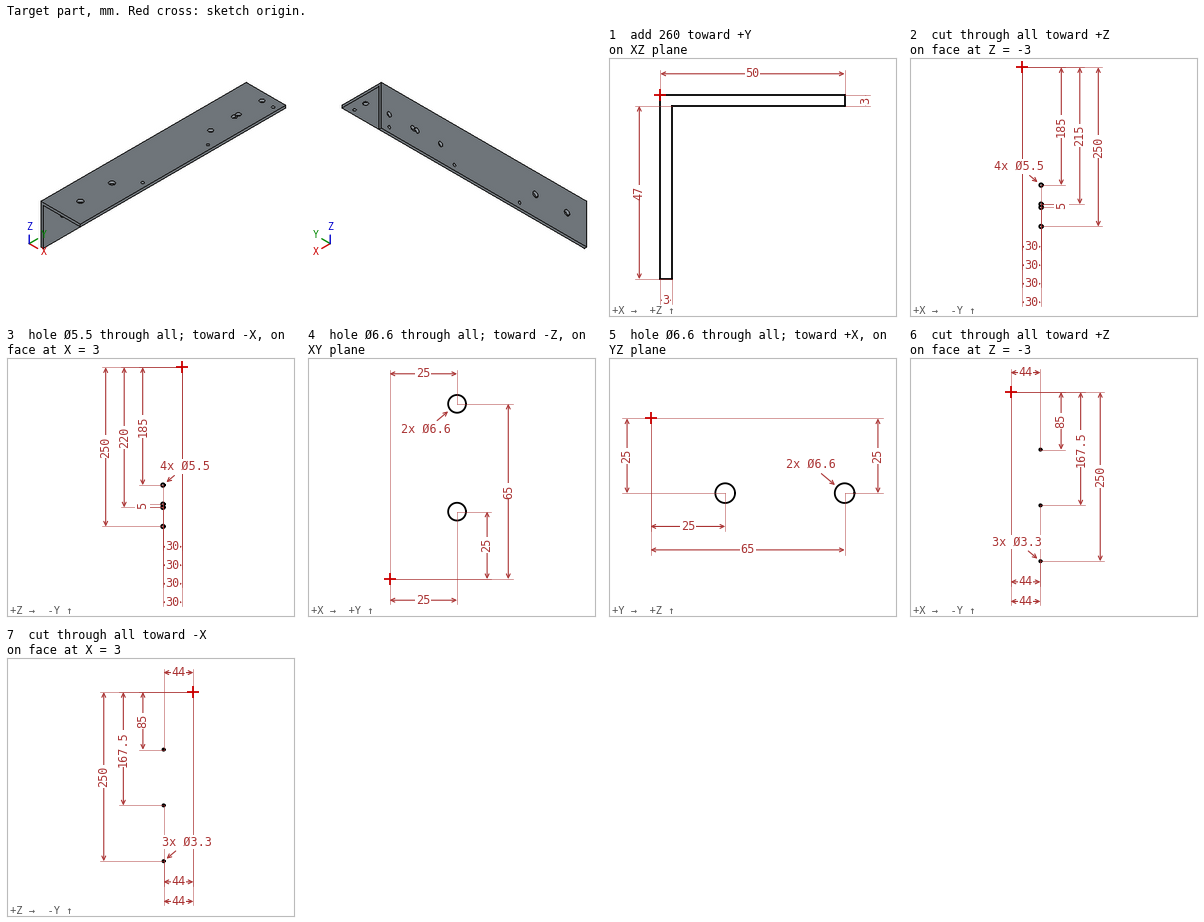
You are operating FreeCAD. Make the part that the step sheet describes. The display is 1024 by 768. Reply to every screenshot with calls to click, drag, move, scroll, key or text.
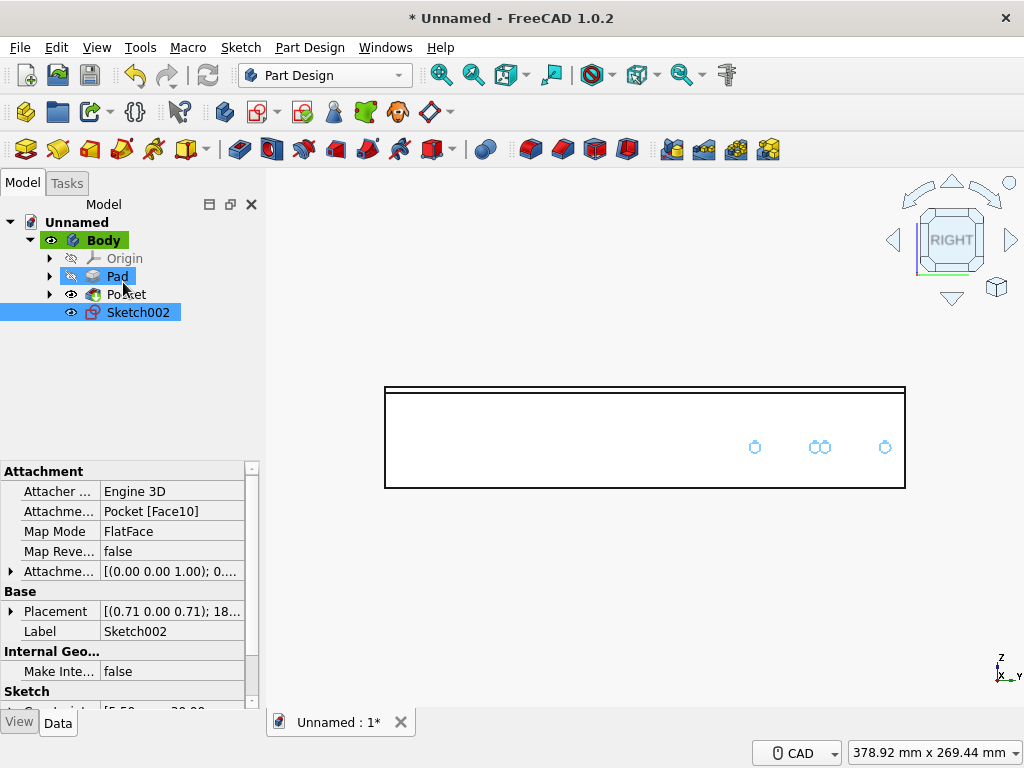
click(272, 150)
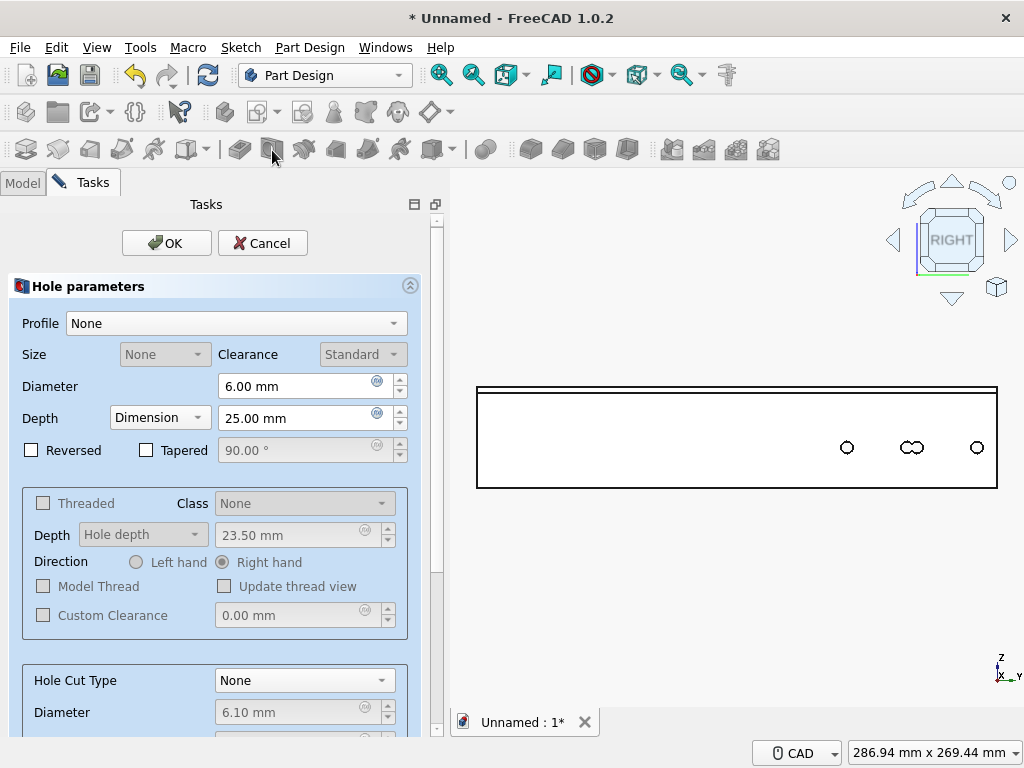
triple_click(305, 386)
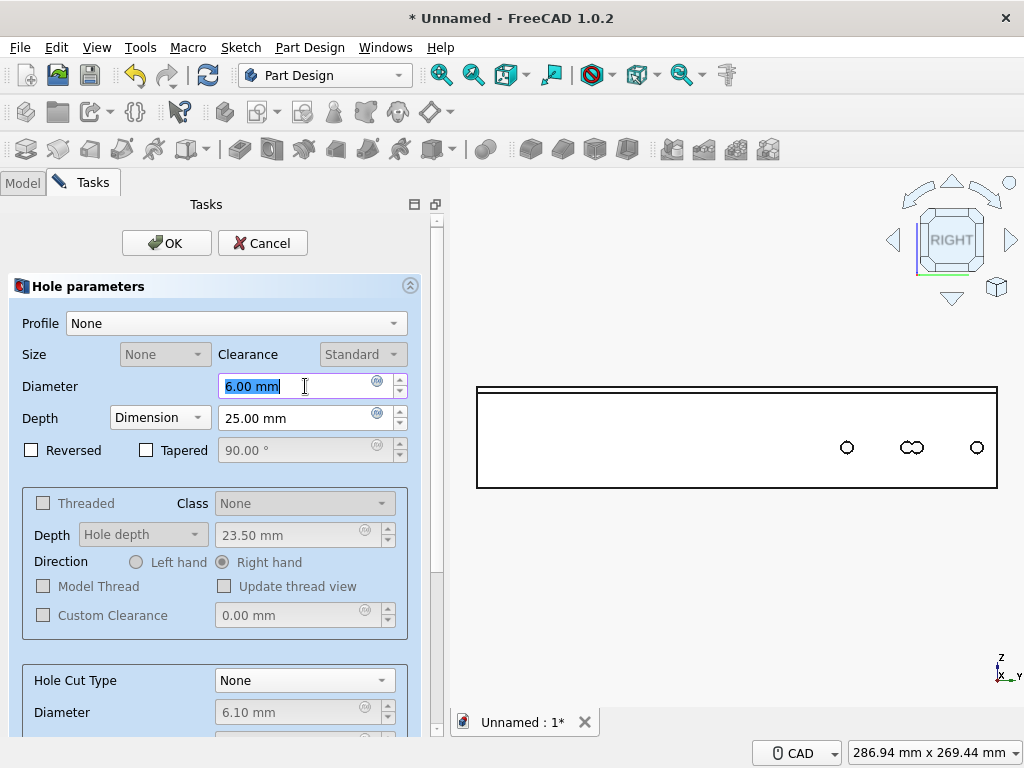
text(5.5)
key(Tab)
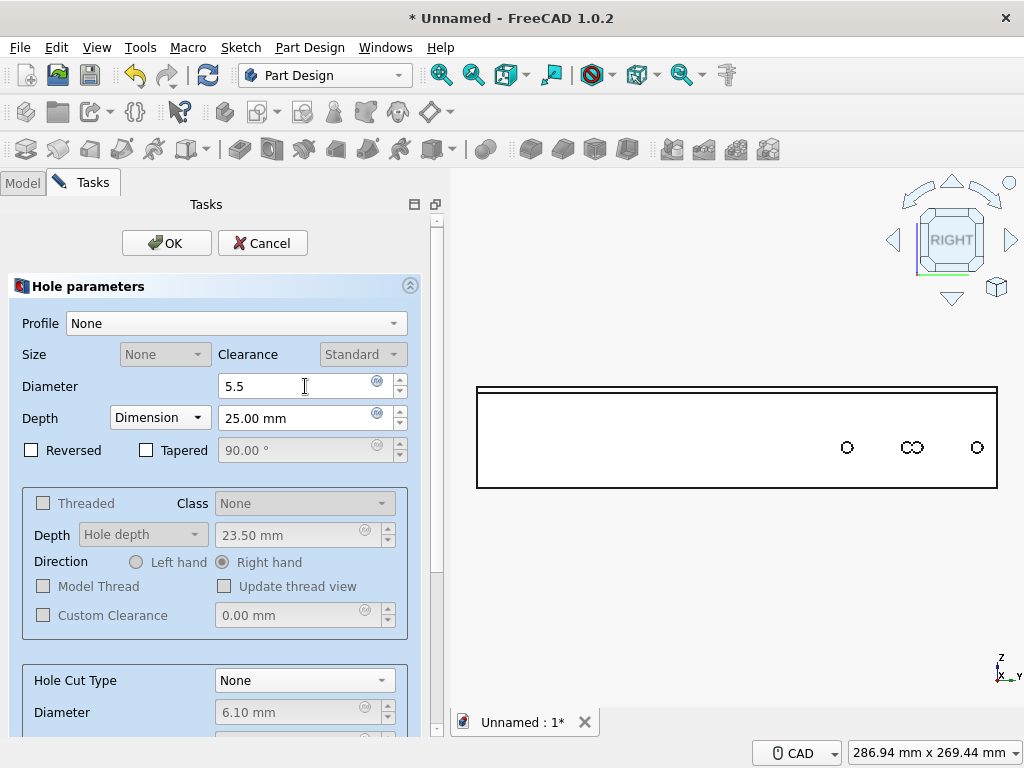
click(161, 418)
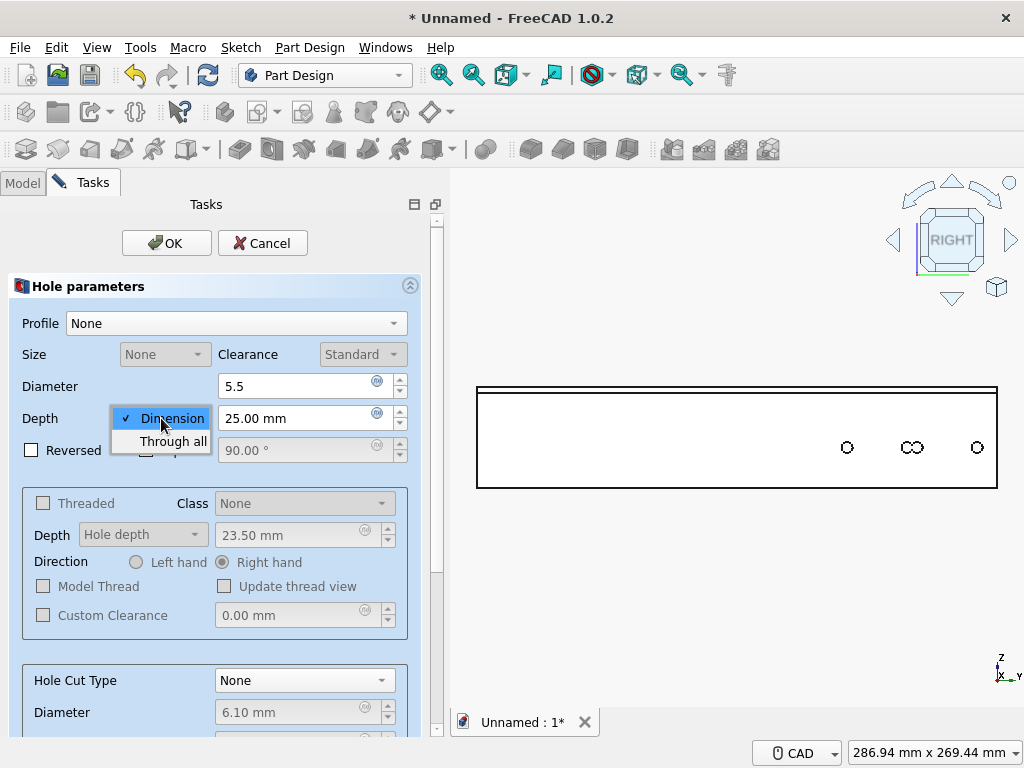
click(160, 442)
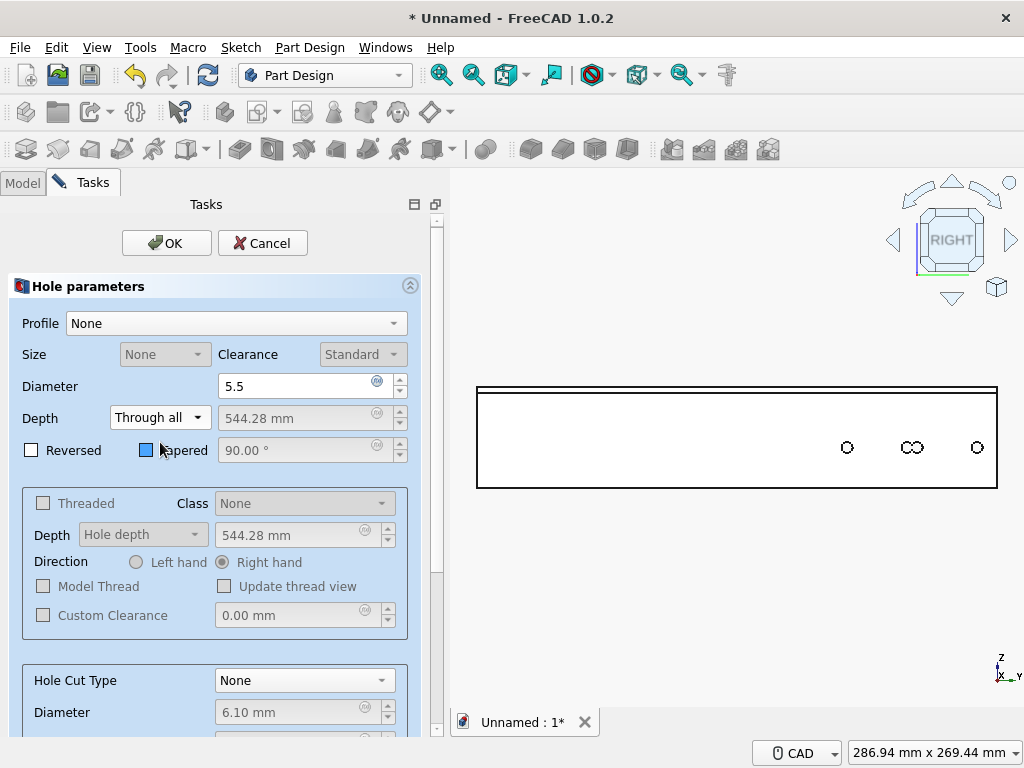
click(167, 243)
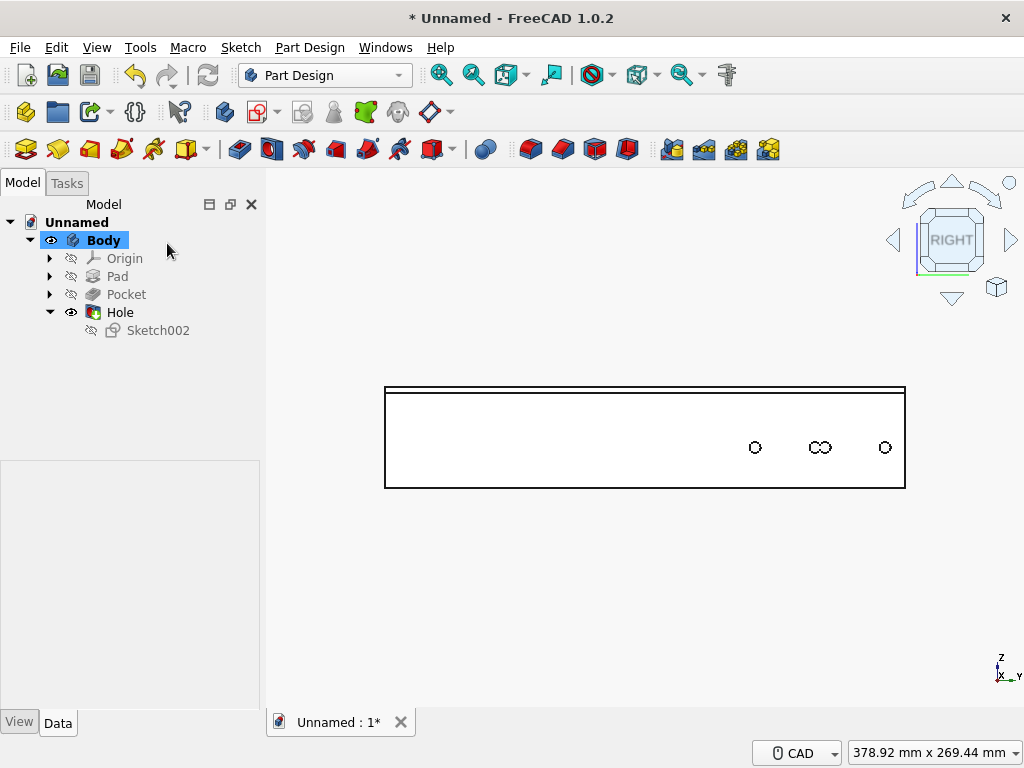
click(258, 112)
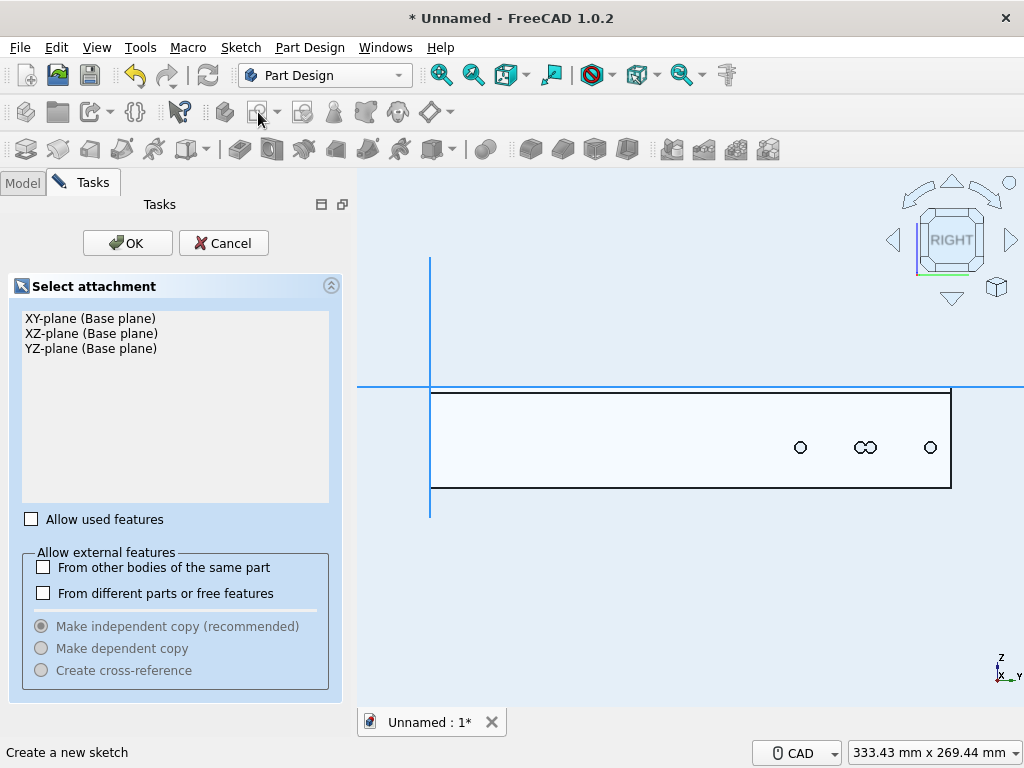
click(82, 318)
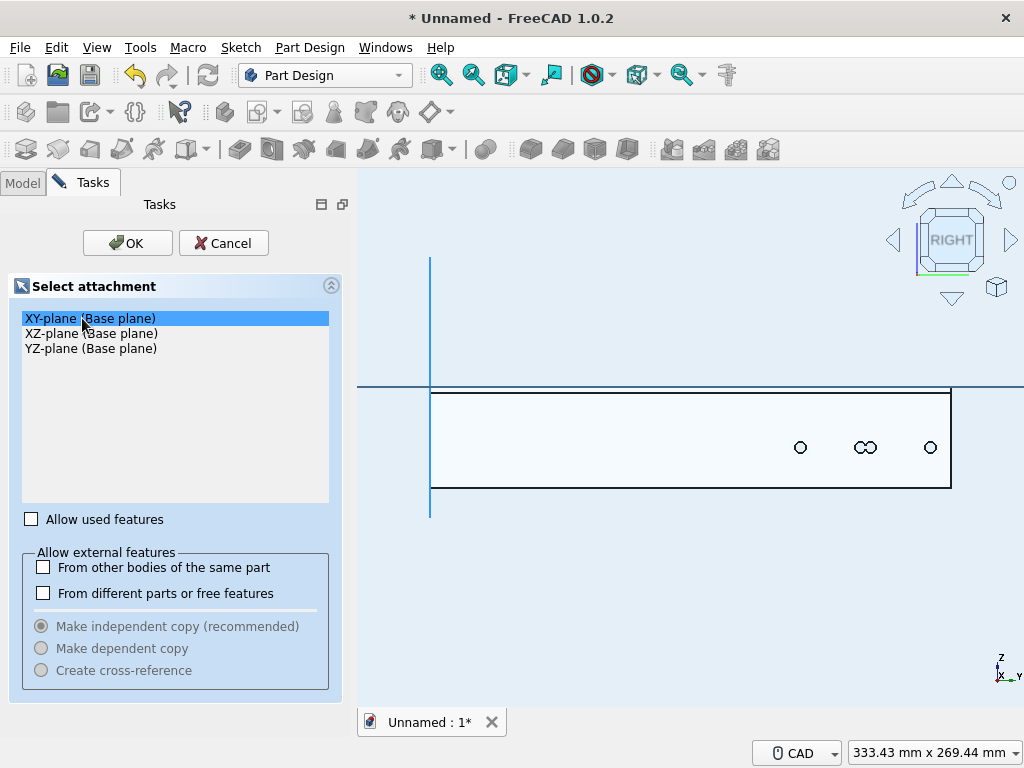
click(128, 243)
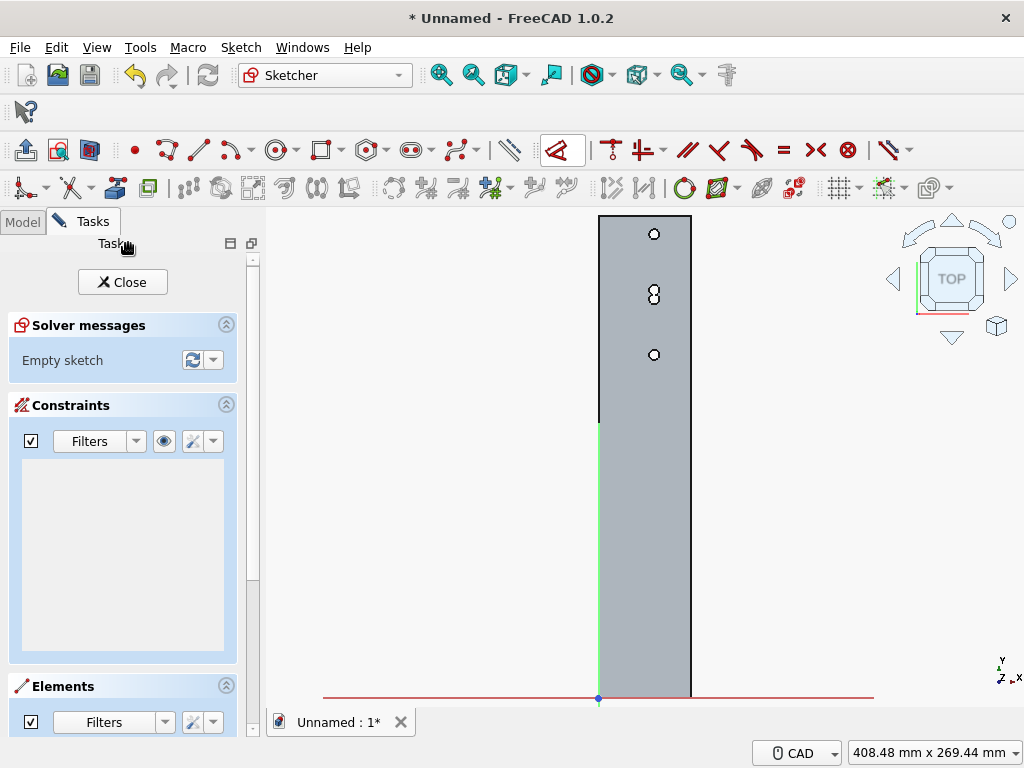
scroll(576, 457, down, 5)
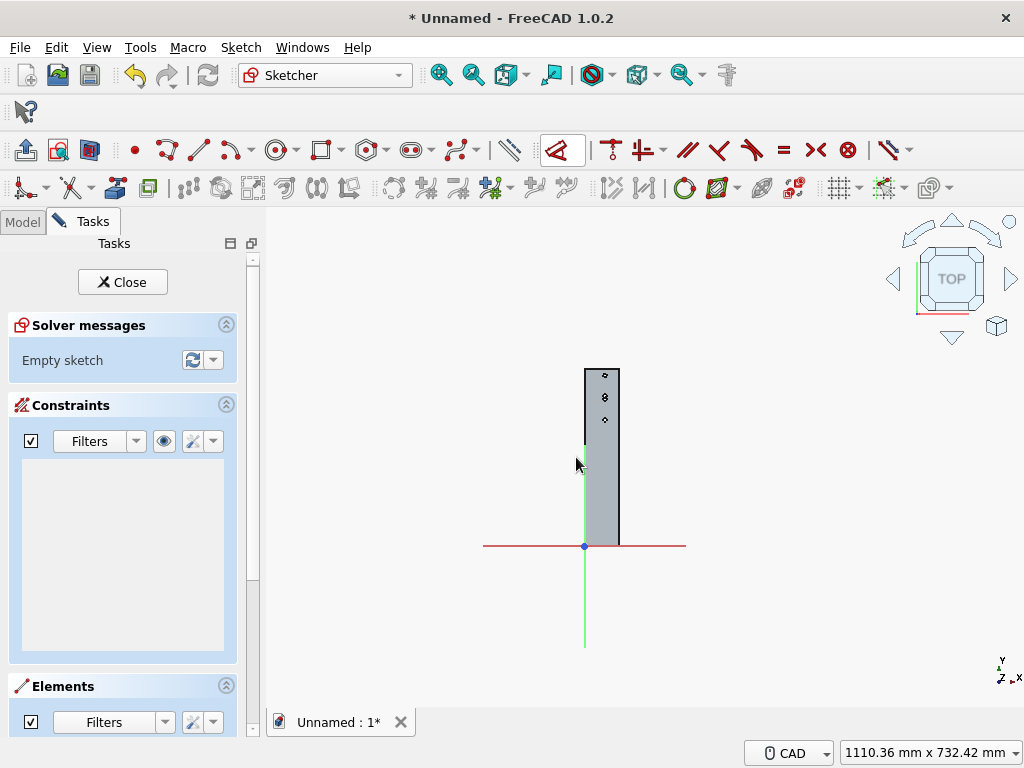
scroll(597, 533, up, 10)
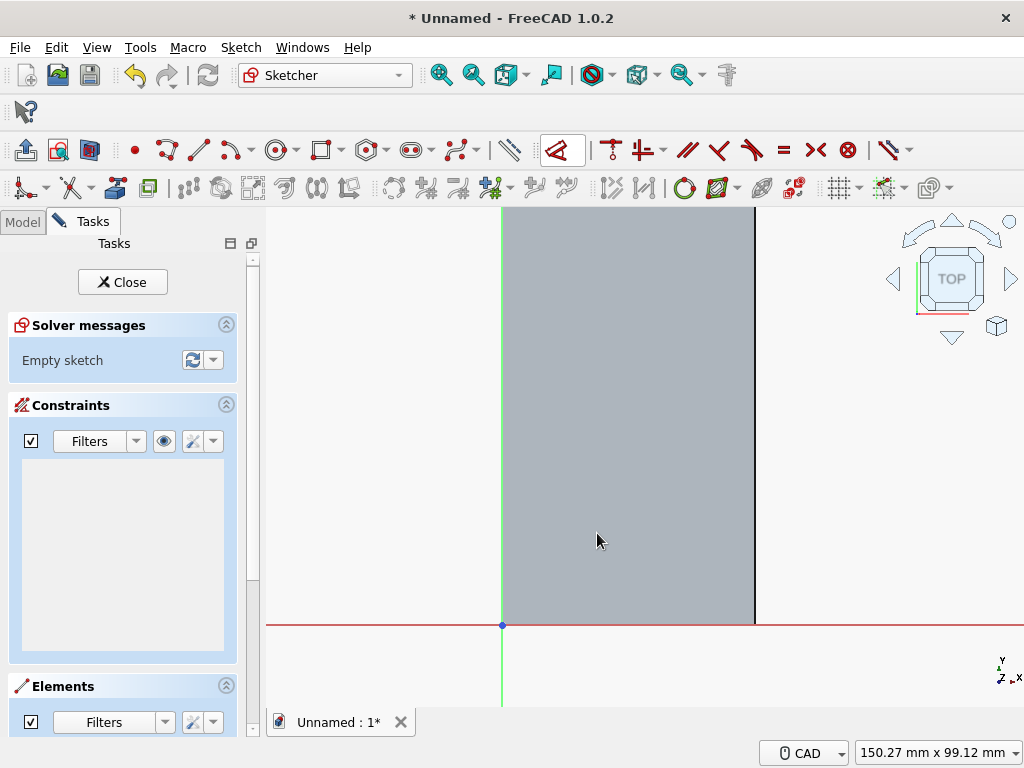
key(g)
key(c)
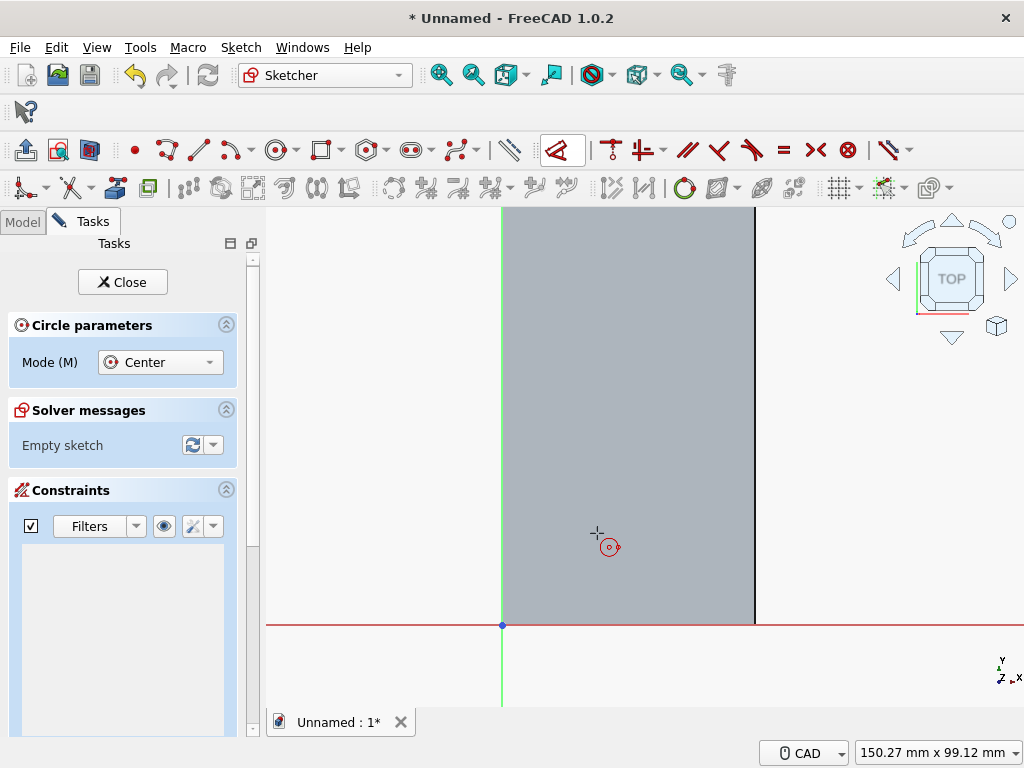
scroll(629, 297, up, 2)